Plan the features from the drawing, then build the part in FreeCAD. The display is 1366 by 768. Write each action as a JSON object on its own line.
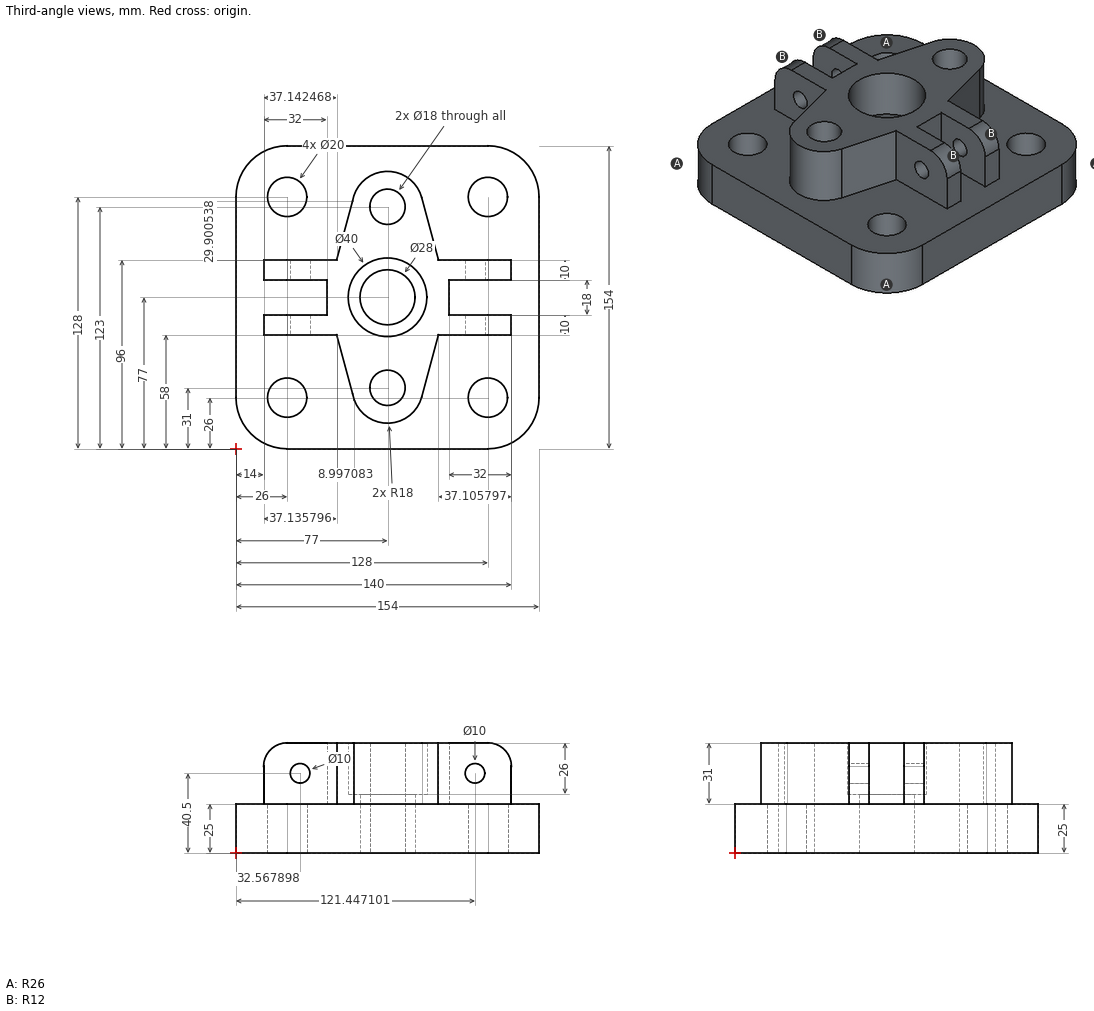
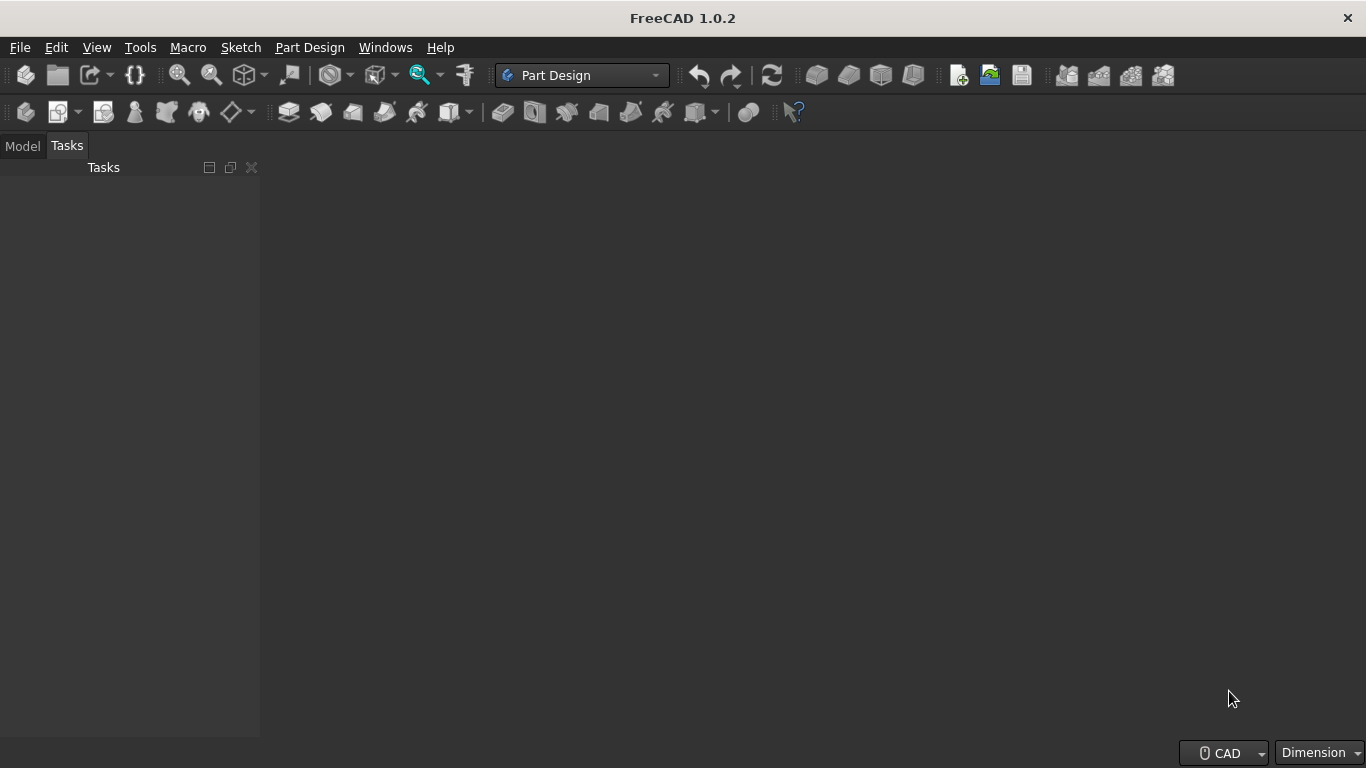
{"action": "left_click", "coordinate": [958, 76]}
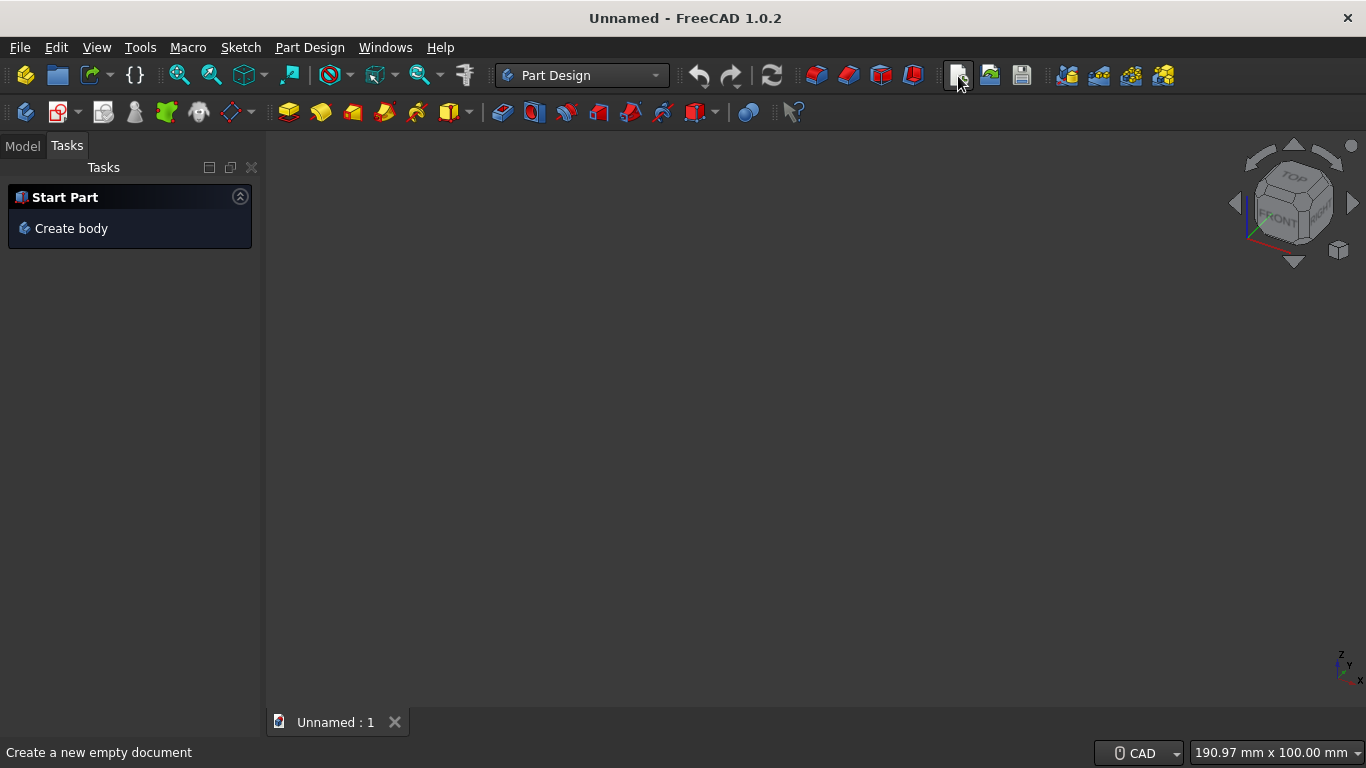
{"action": "left_click", "coordinate": [58, 112]}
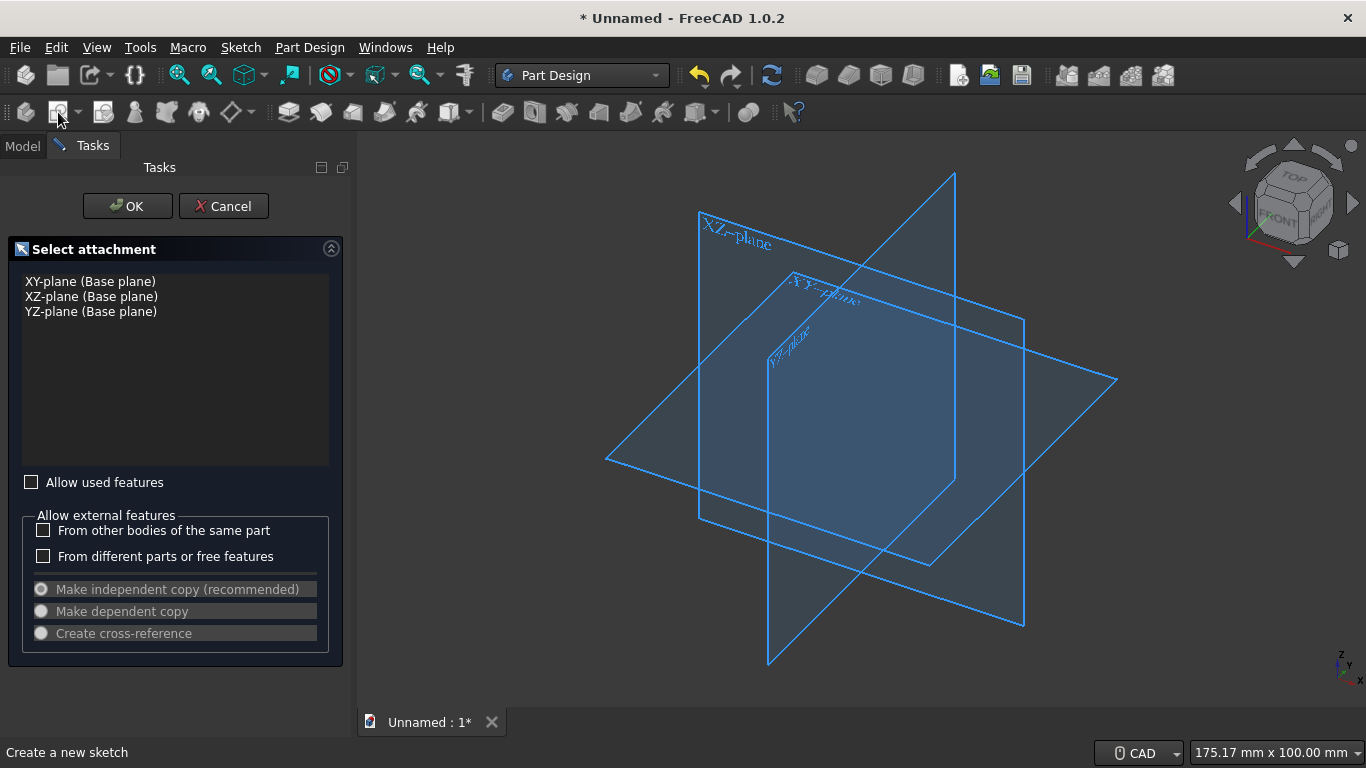
{"action": "left_click", "coordinate": [82, 282]}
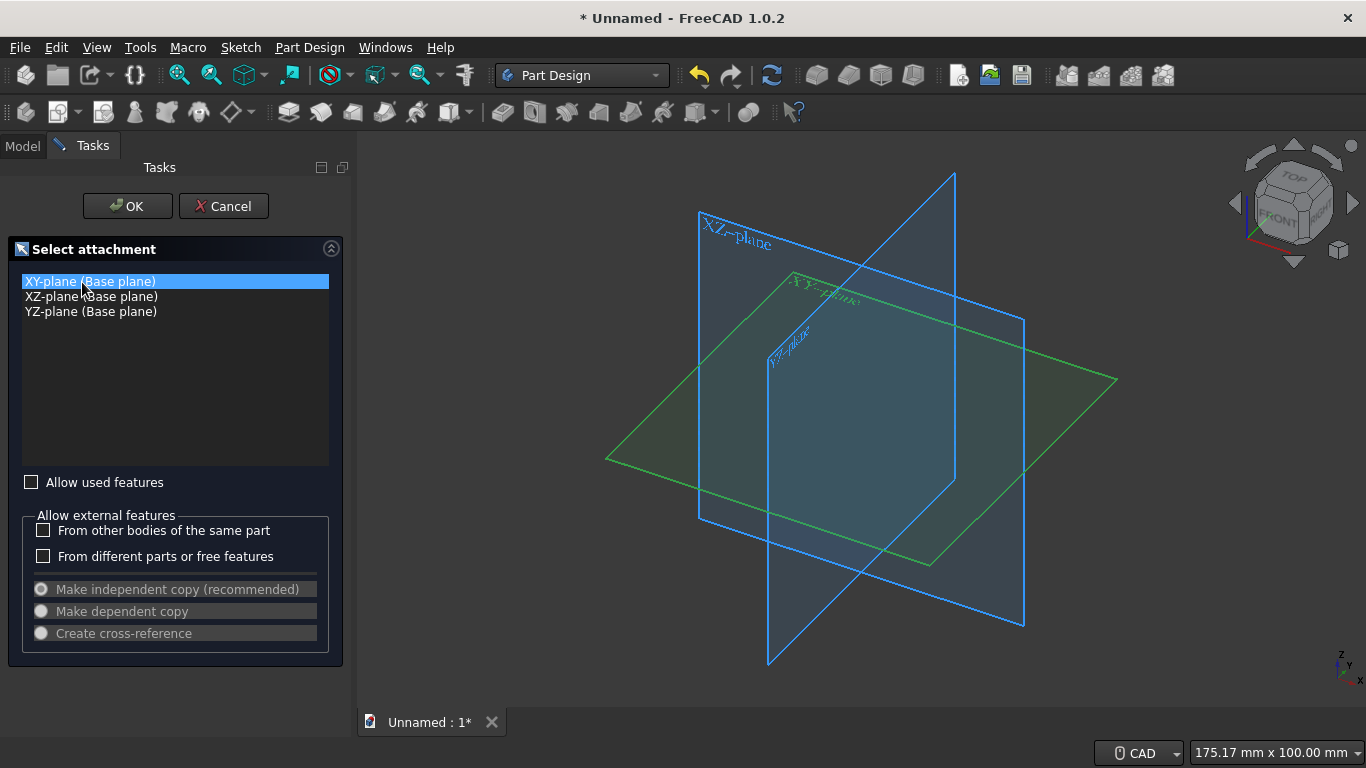
{"action": "left_click", "coordinate": [128, 206]}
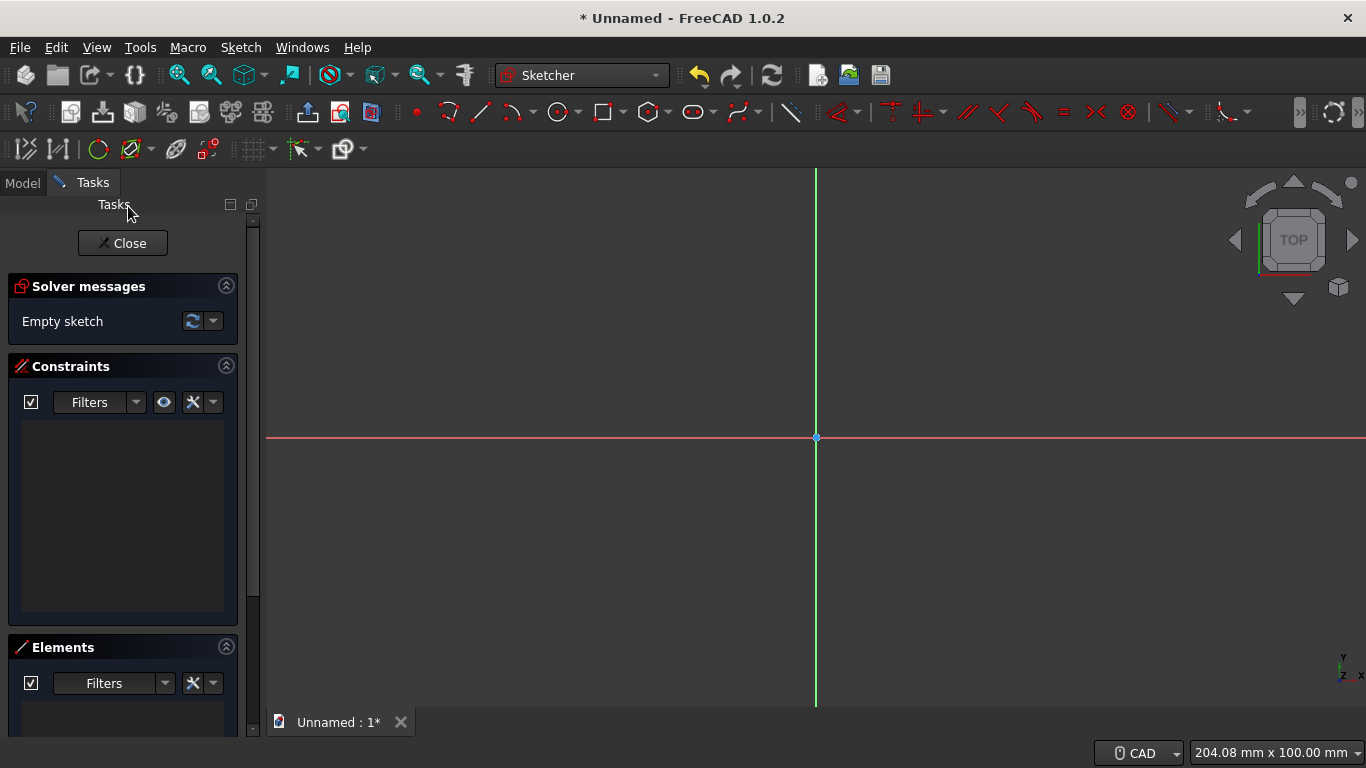
{"action": "scroll", "coordinate": [466, 679], "scroll_direction": "down", "scroll_amount": 5}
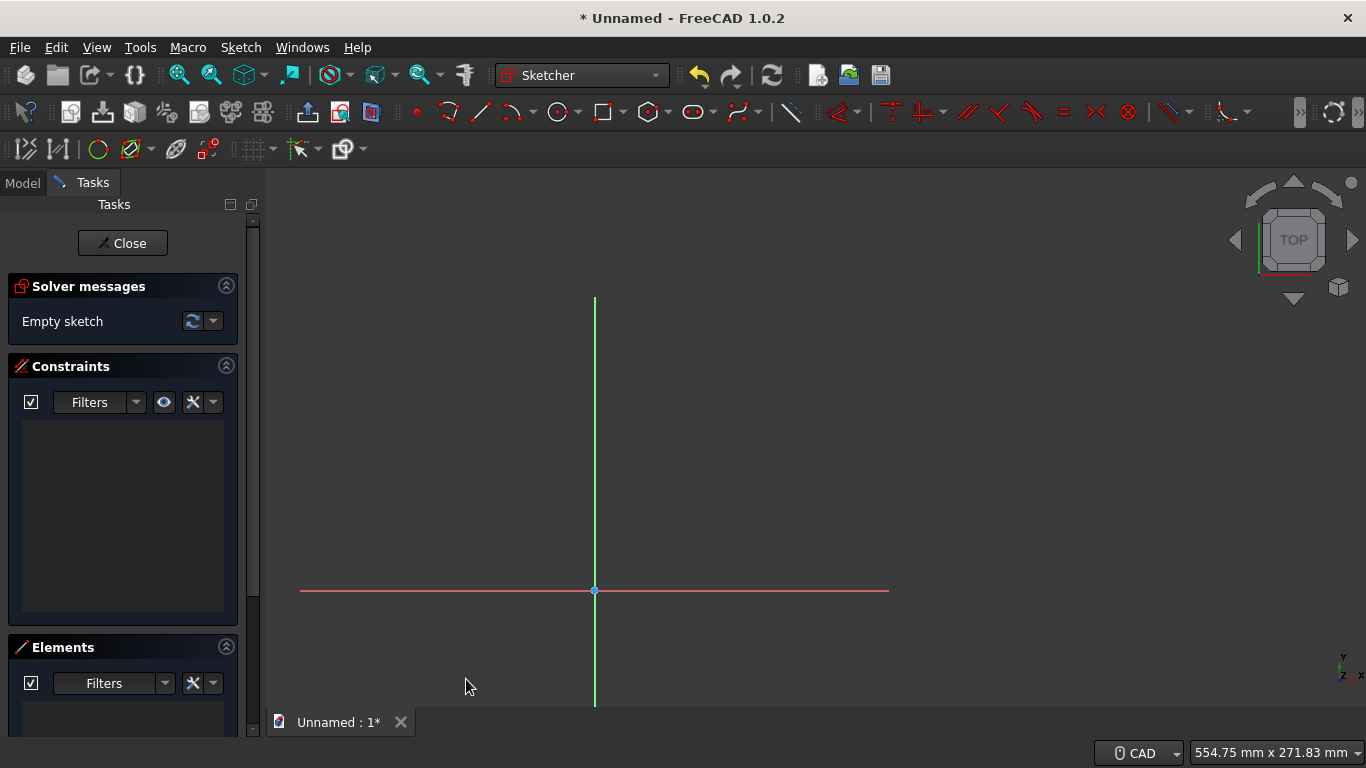
{"action": "left_click", "coordinate": [604, 112]}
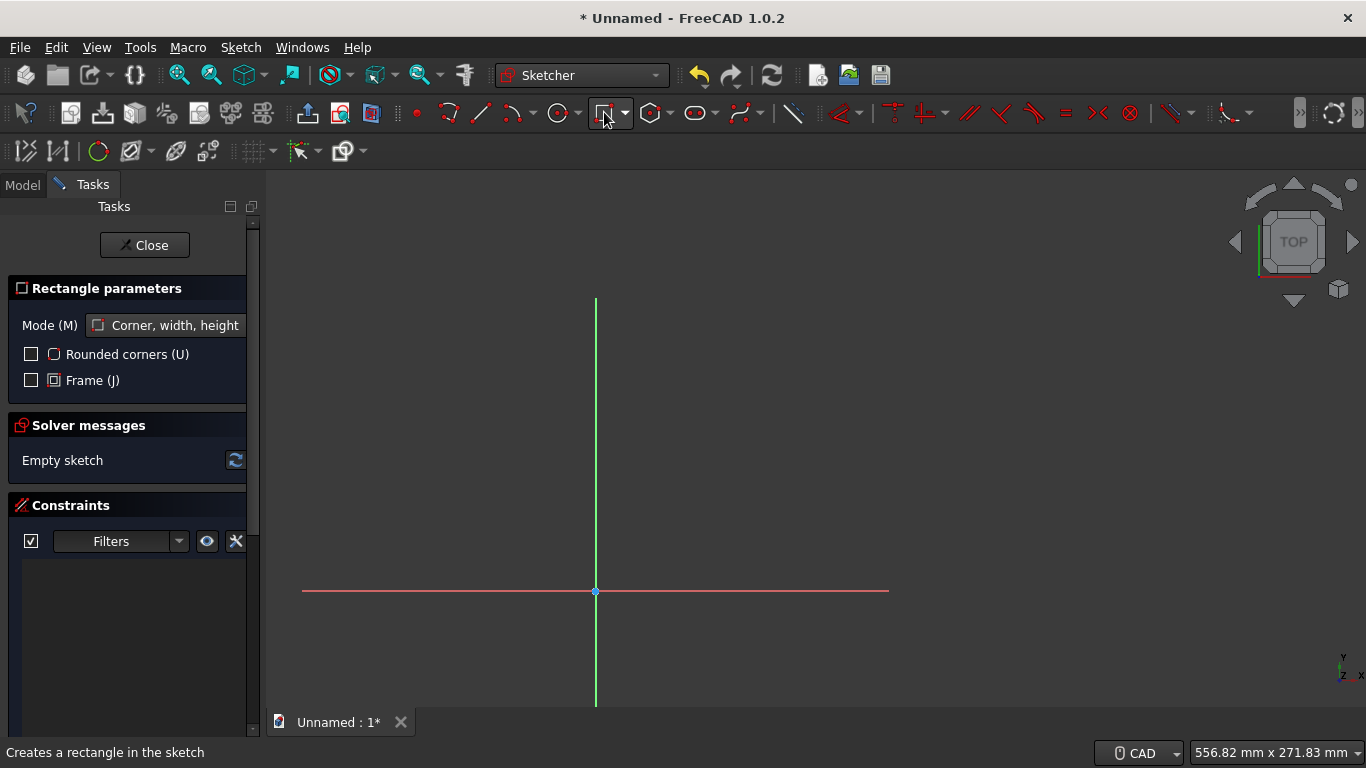
{"action": "left_click", "coordinate": [596, 591]}
{"action": "left_click", "coordinate": [900, 287]}
{"action": "key", "text": "Escape"}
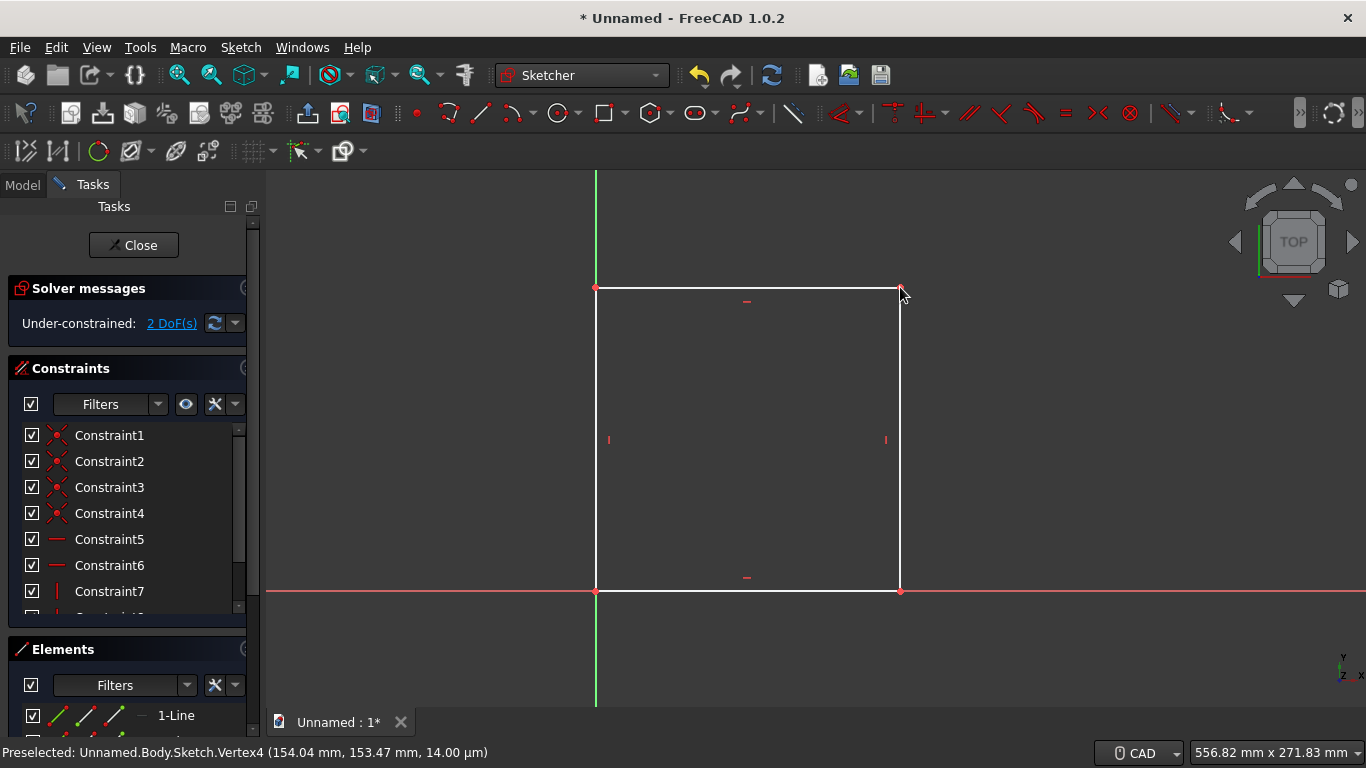
{"action": "left_click", "coordinate": [687, 591]}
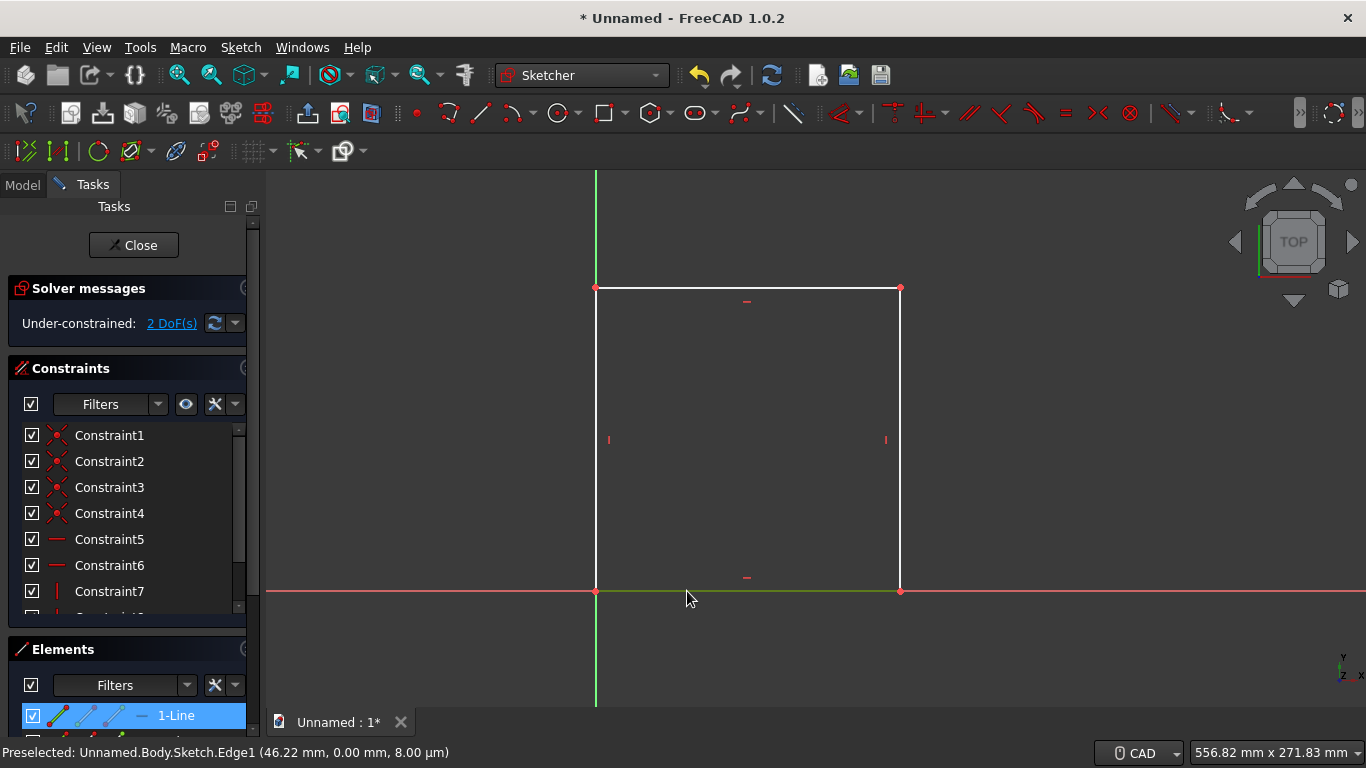
{"action": "key", "text": "l"}